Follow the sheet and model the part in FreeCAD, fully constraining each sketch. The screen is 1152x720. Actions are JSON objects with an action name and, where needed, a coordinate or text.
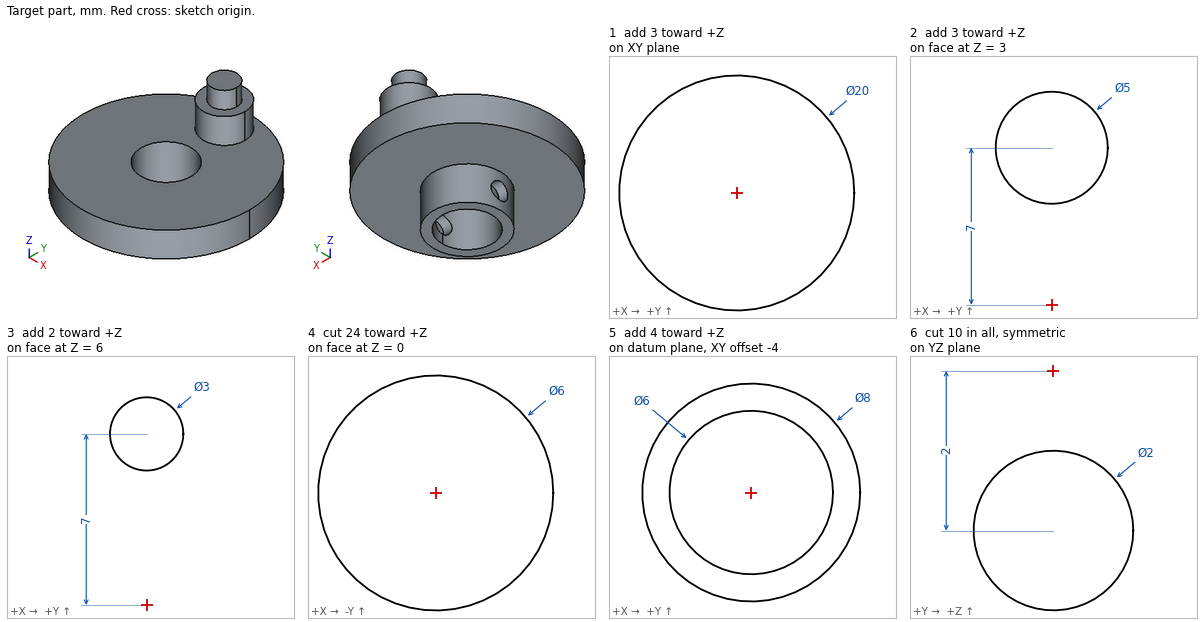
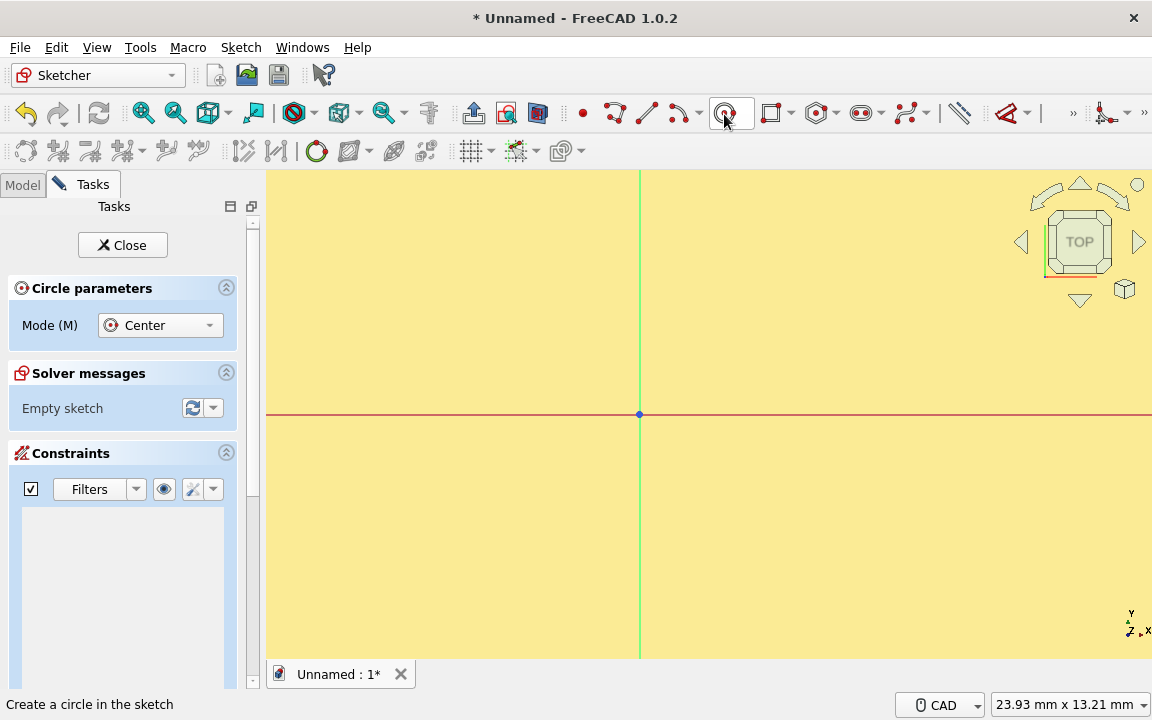
{"action": "left_click", "coordinate": [640, 414]}
{"action": "left_click", "coordinate": [744, 310]}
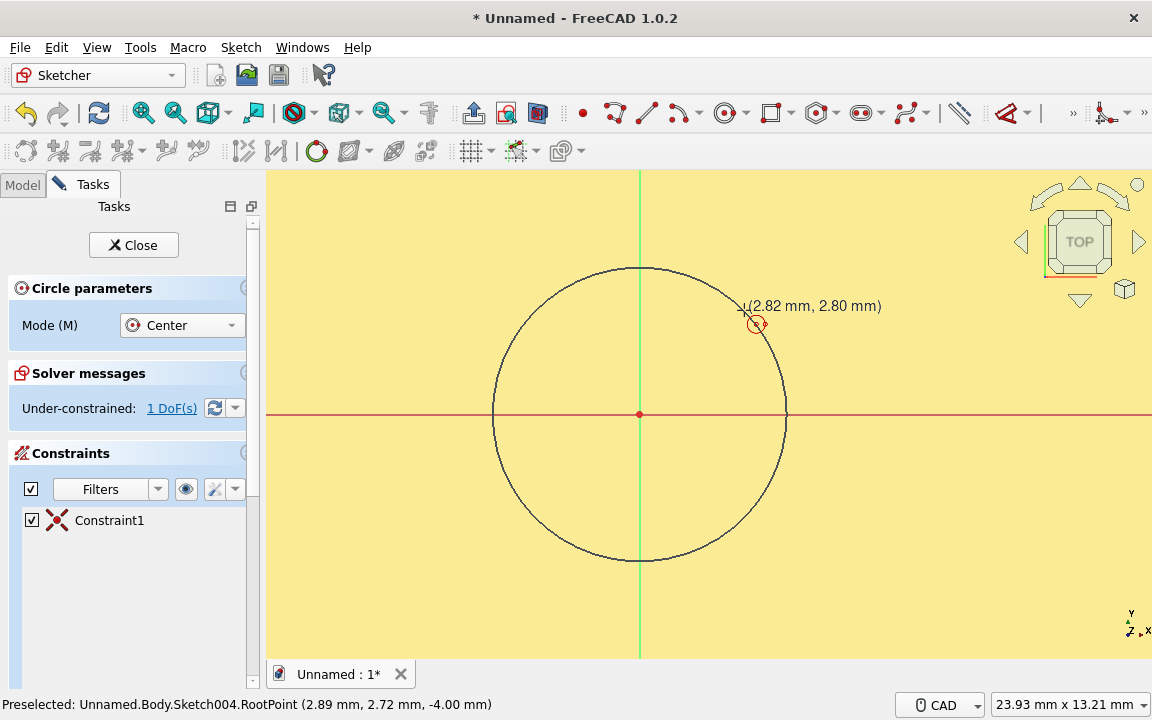
{"action": "left_click", "coordinate": [640, 414]}
{"action": "left_click", "coordinate": [718, 336]}
{"action": "key", "text": "Escape"}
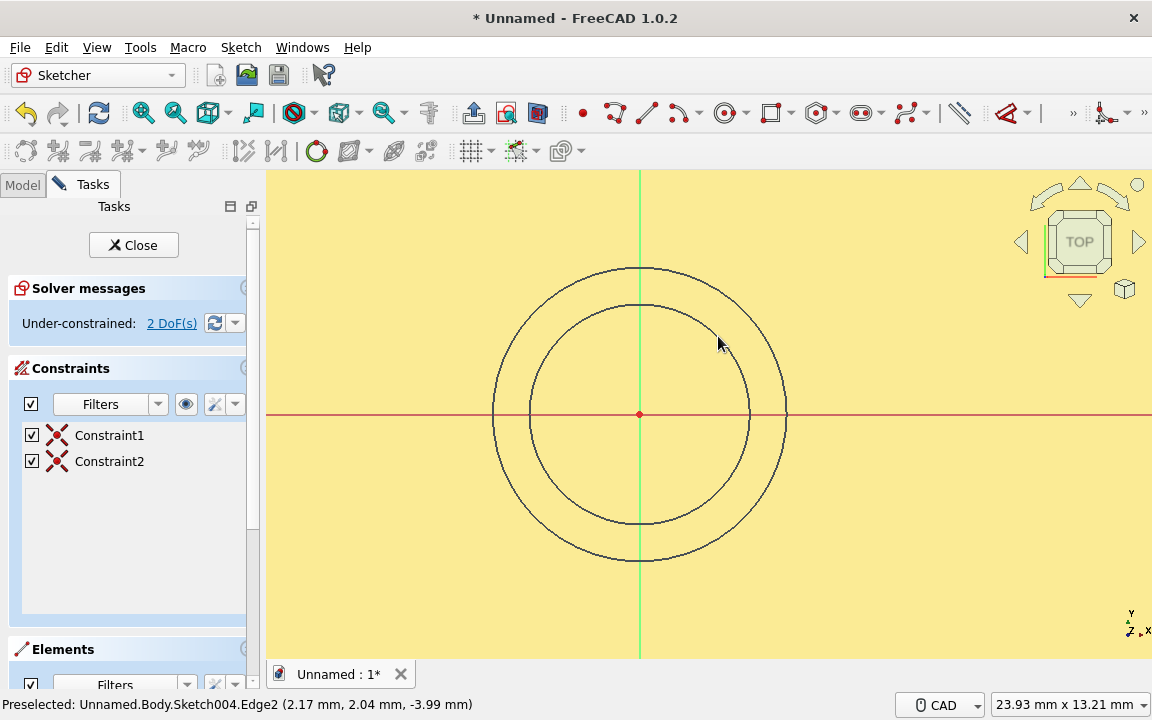
{"action": "key", "text": "d"}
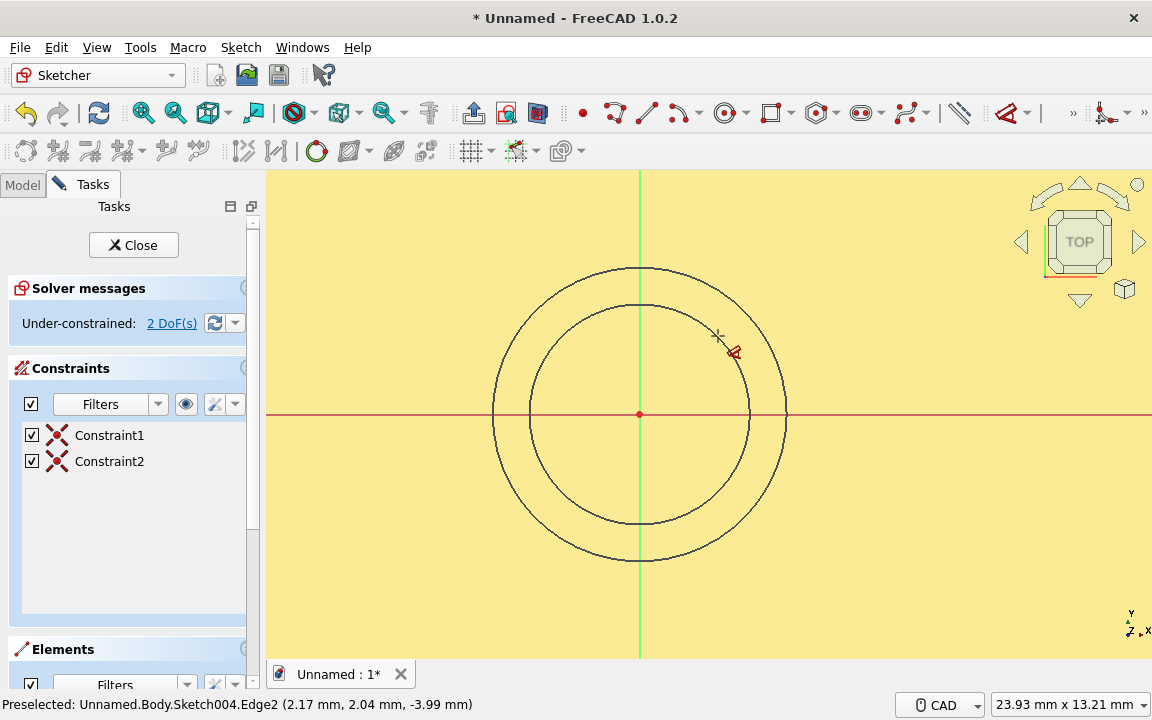
{"action": "left_click", "coordinate": [743, 310]}
{"action": "left_click", "coordinate": [765, 287]}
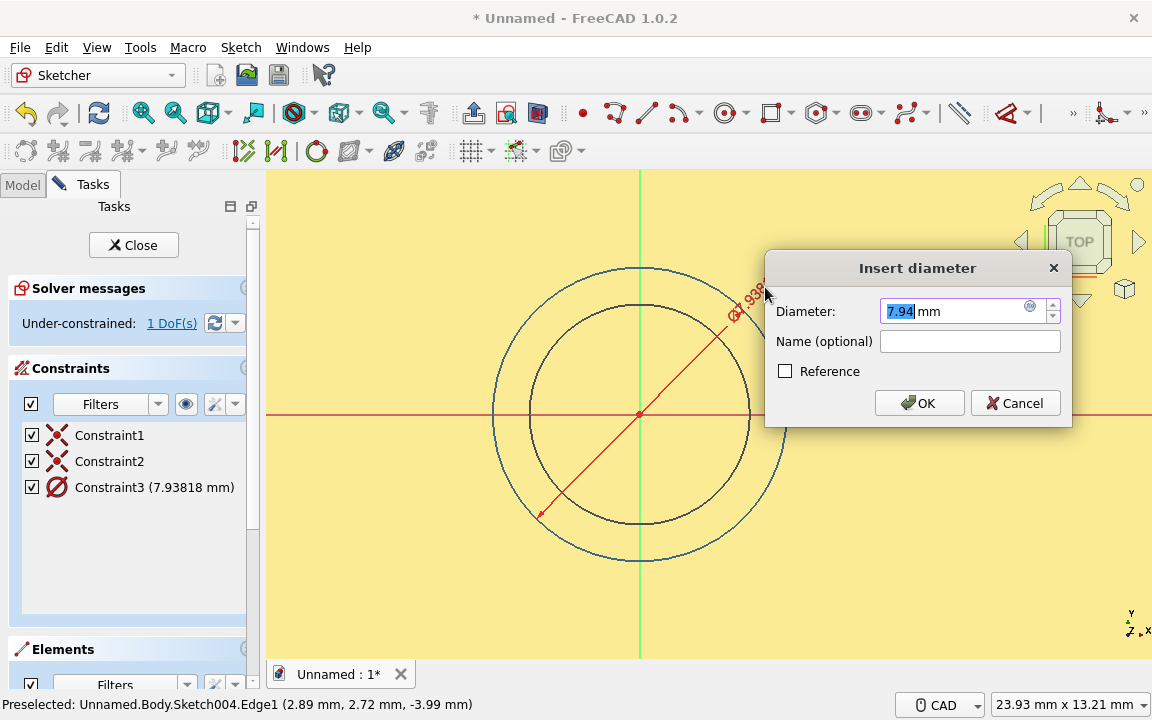
{"action": "type", "text": "8"}
{"action": "key", "text": "Return"}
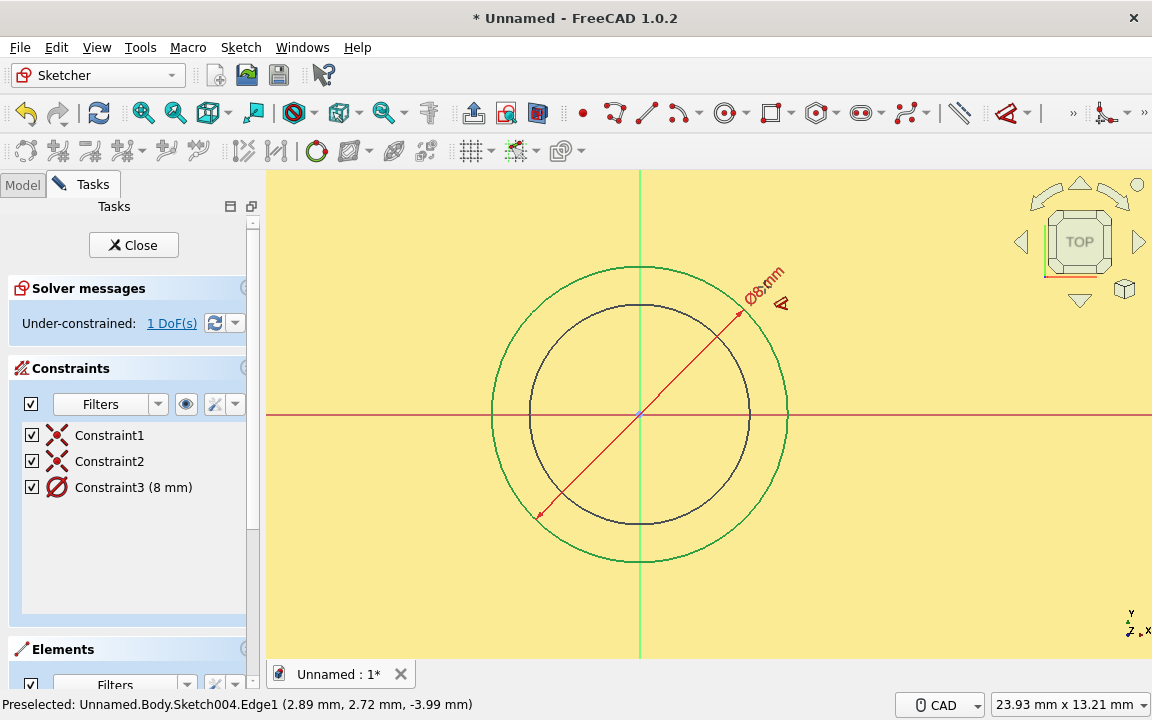
{"action": "left_click", "coordinate": [717, 336]}
{"action": "left_click", "coordinate": [798, 367]}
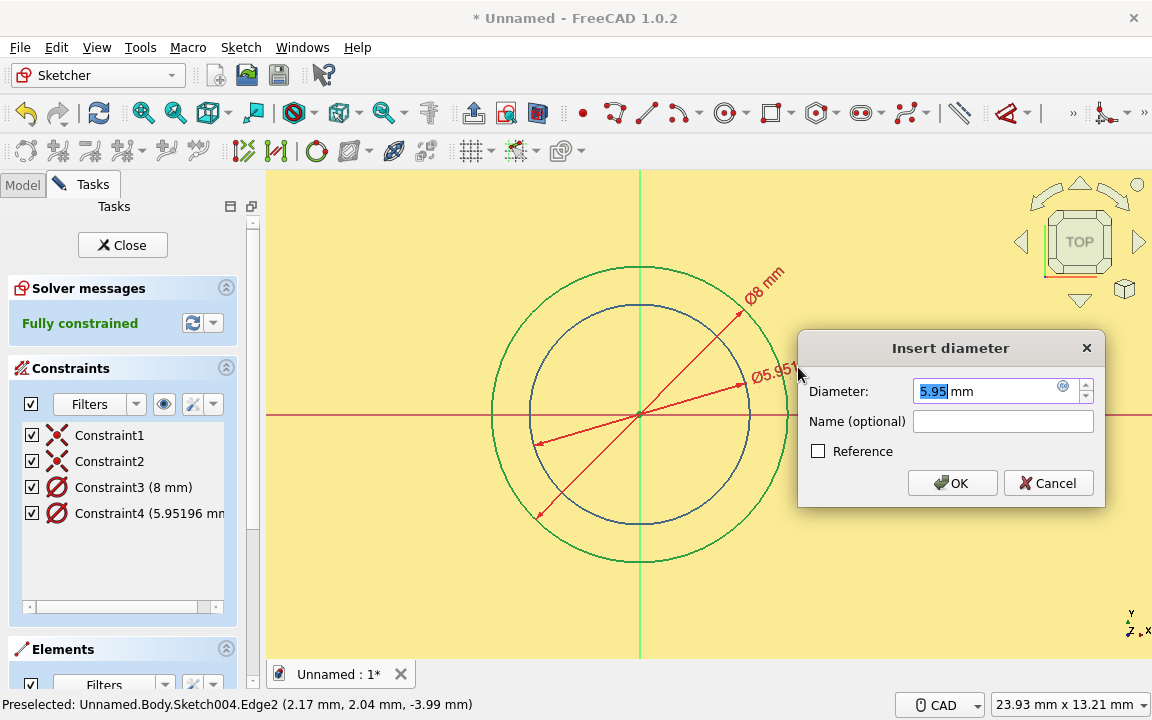
{"action": "type", "text": "6"}
{"action": "key", "text": "Return"}
{"action": "key", "text": "Escape"}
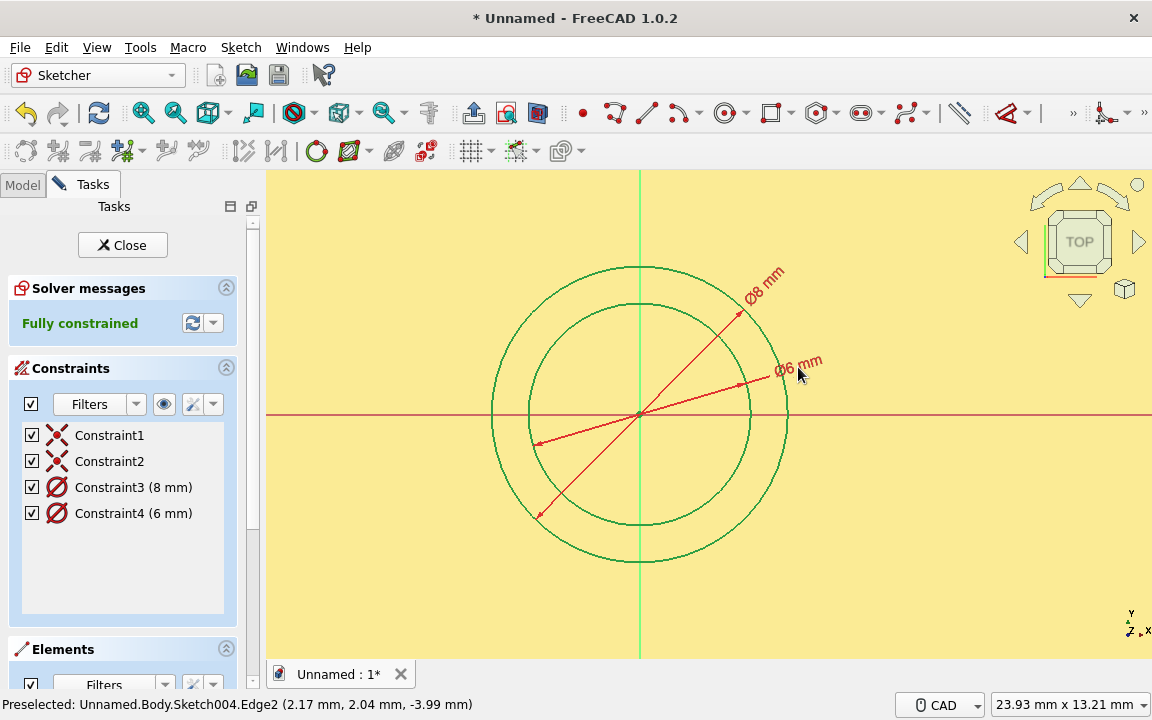
{"action": "left_click", "coordinate": [123, 245]}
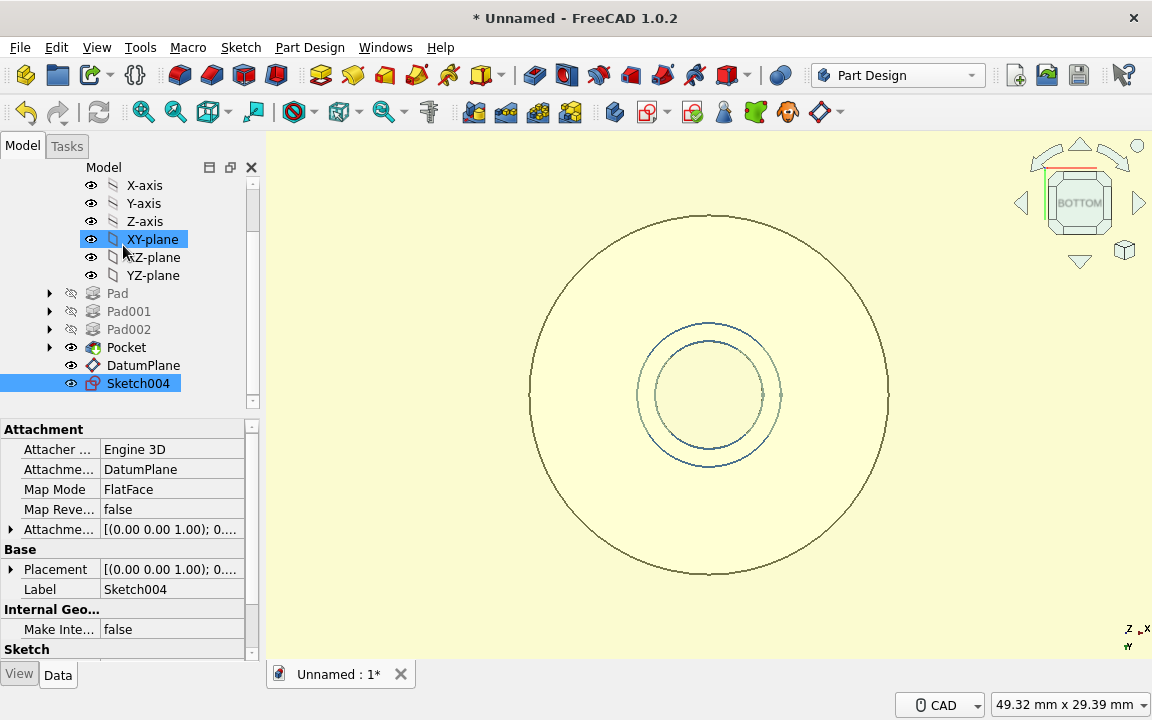
{"action": "left_click", "coordinate": [322, 76]}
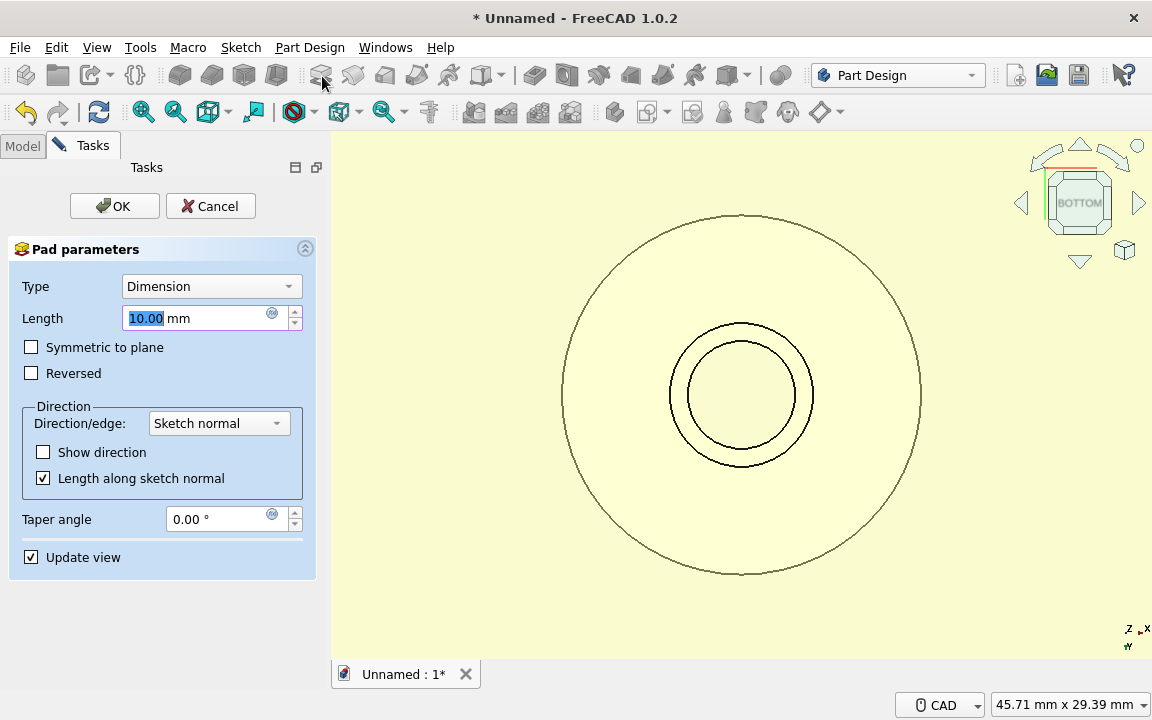
{"action": "type", "text": "4"}
{"action": "key", "text": "Tab"}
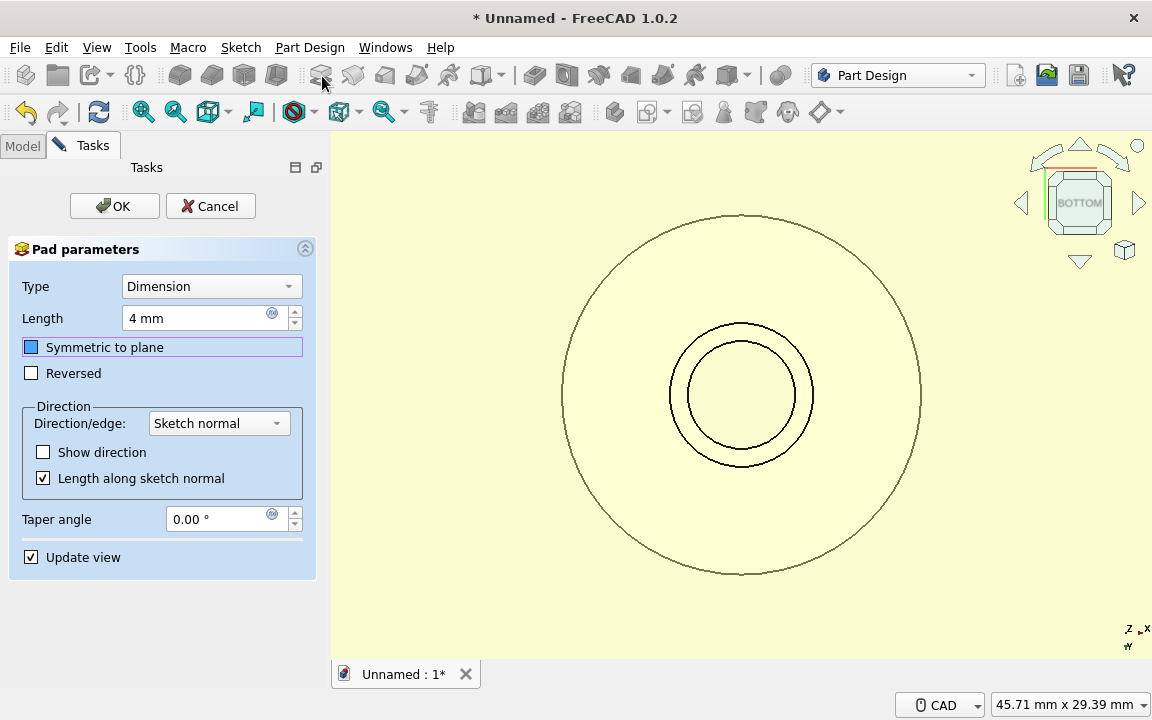
{"action": "left_click", "coordinate": [115, 206]}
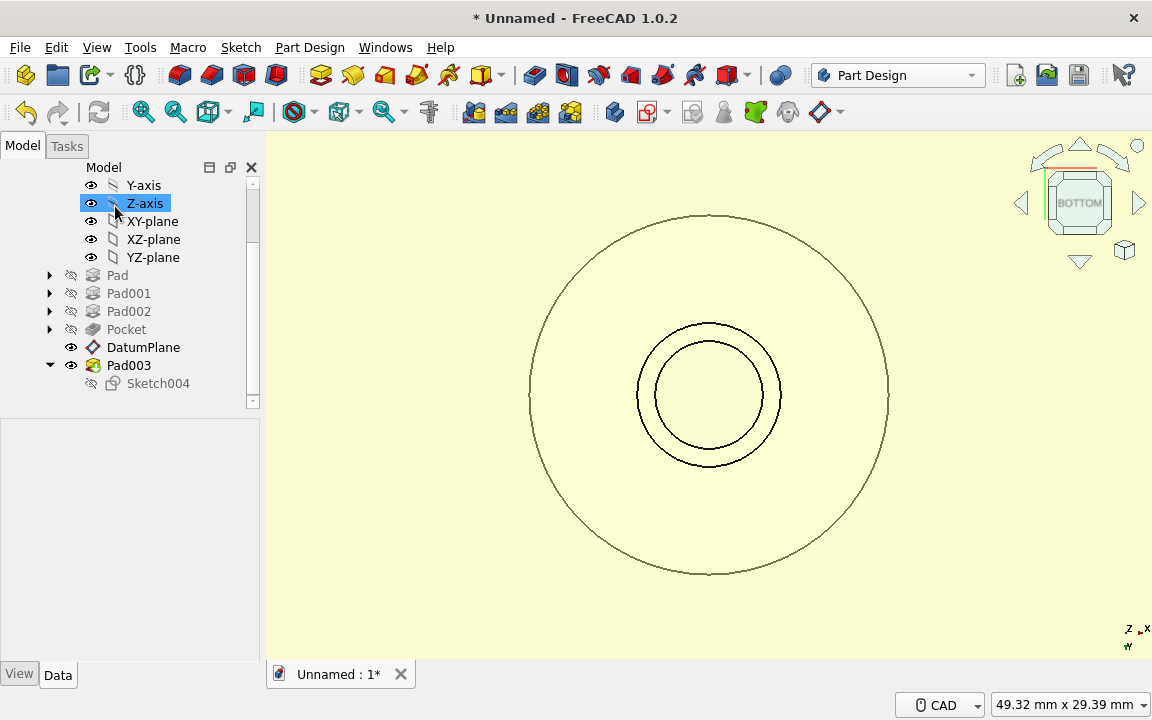
{"action": "left_click", "coordinate": [116, 347]}
{"action": "key", "text": "space"}